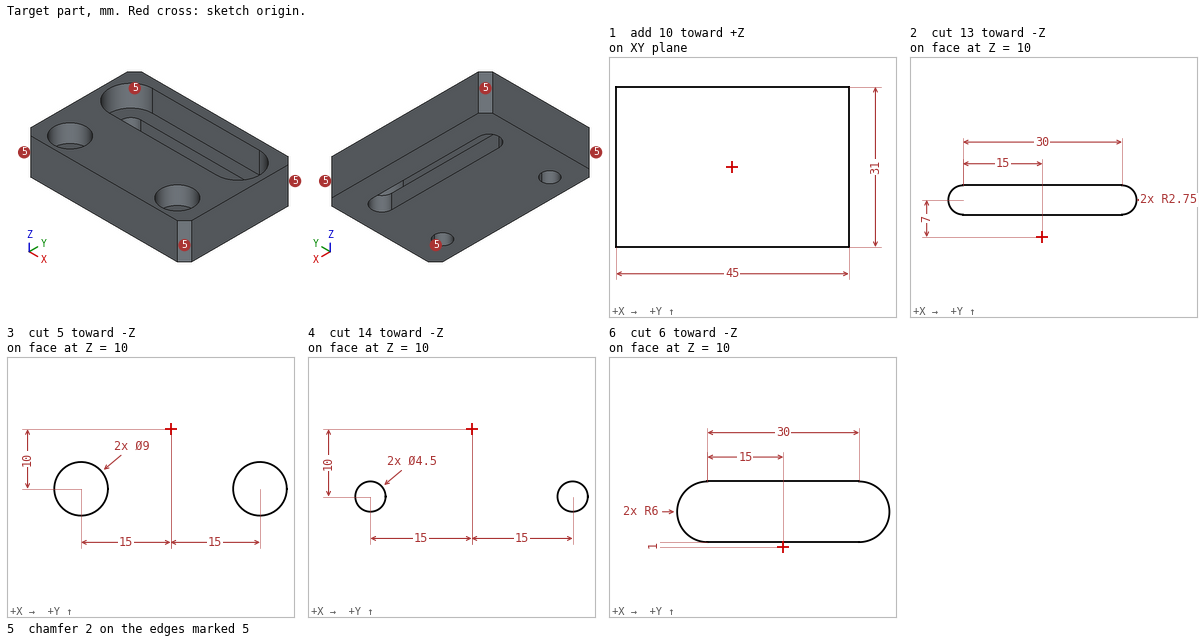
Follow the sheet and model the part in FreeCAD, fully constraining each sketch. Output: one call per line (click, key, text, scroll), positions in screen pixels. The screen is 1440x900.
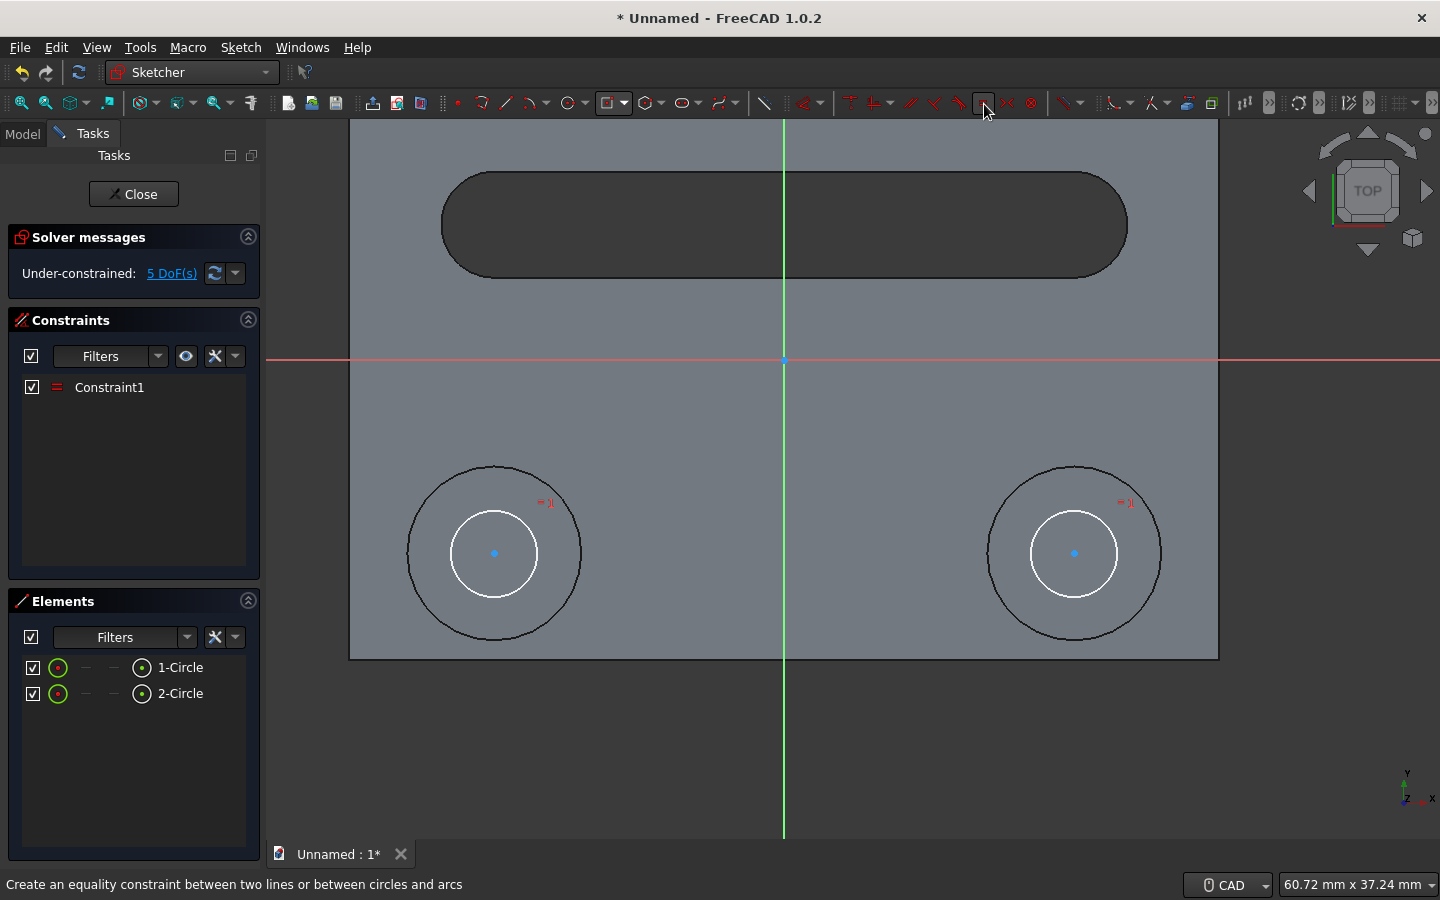
click(494, 554)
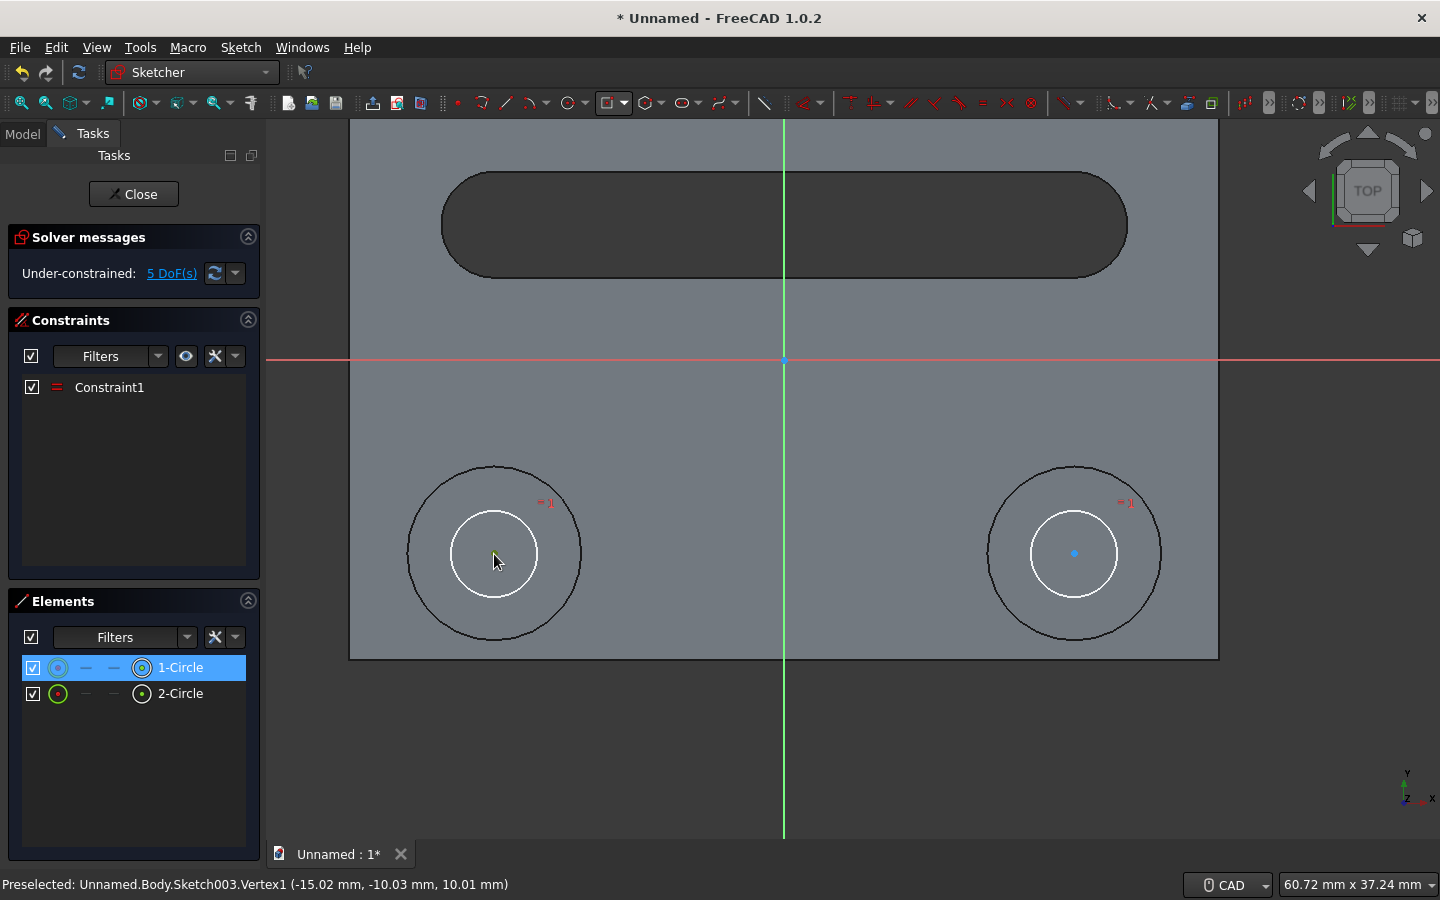
click(1074, 554)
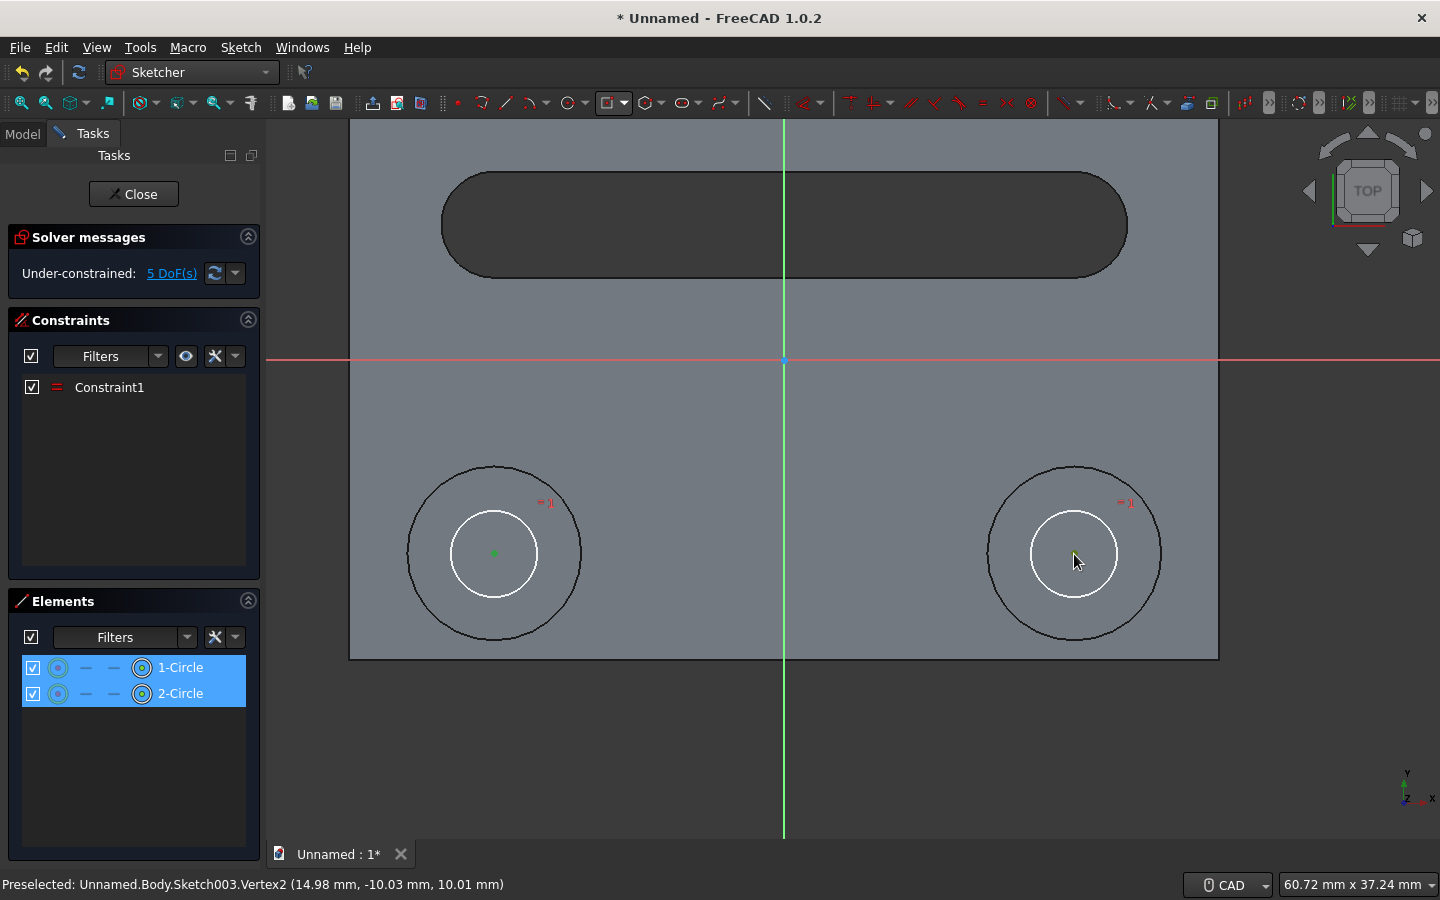
key(h)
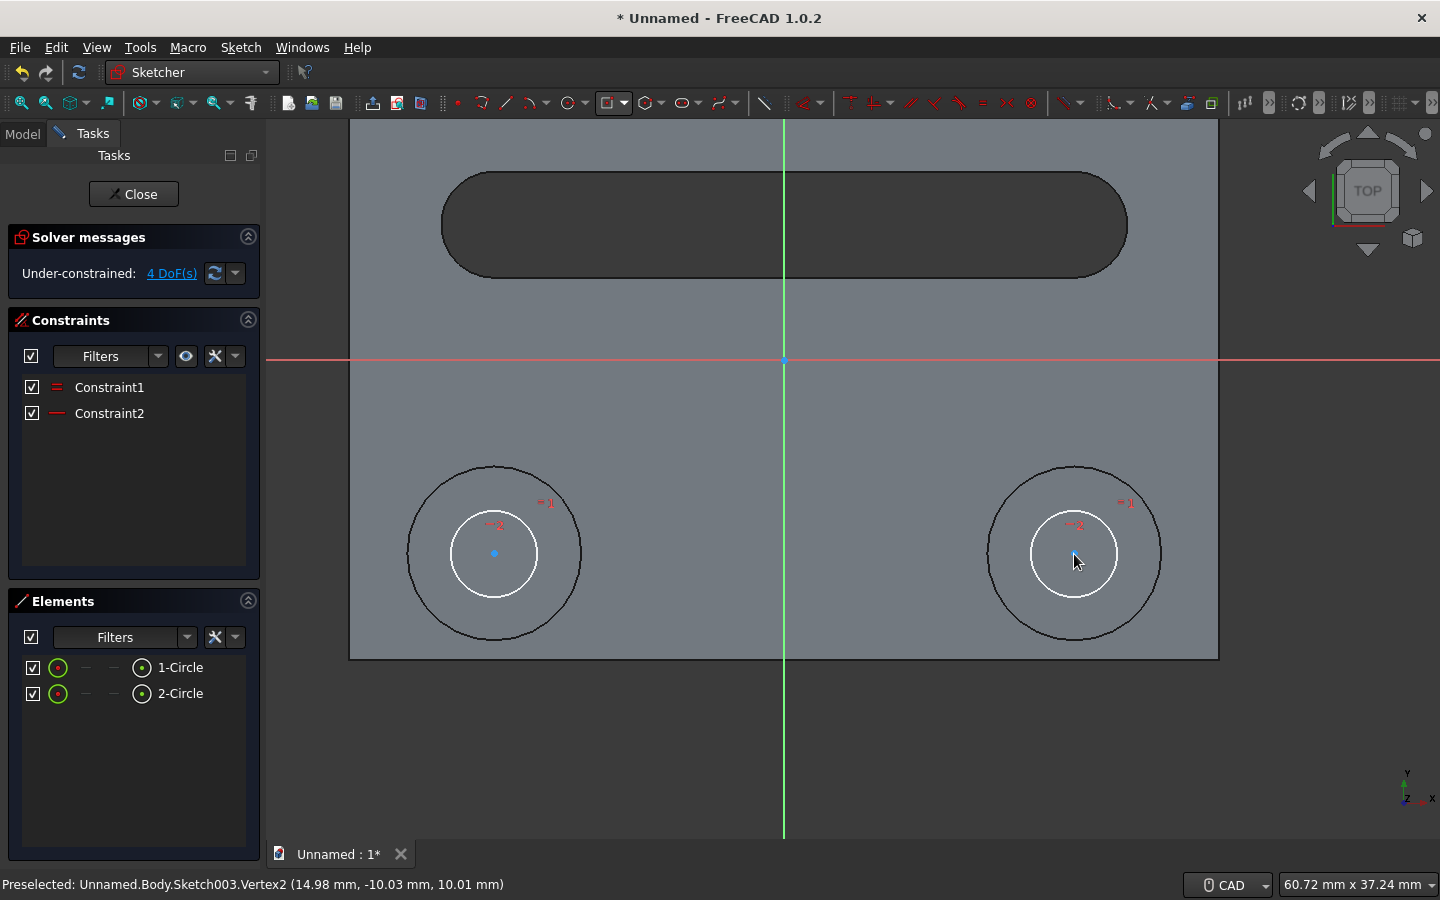
click(804, 104)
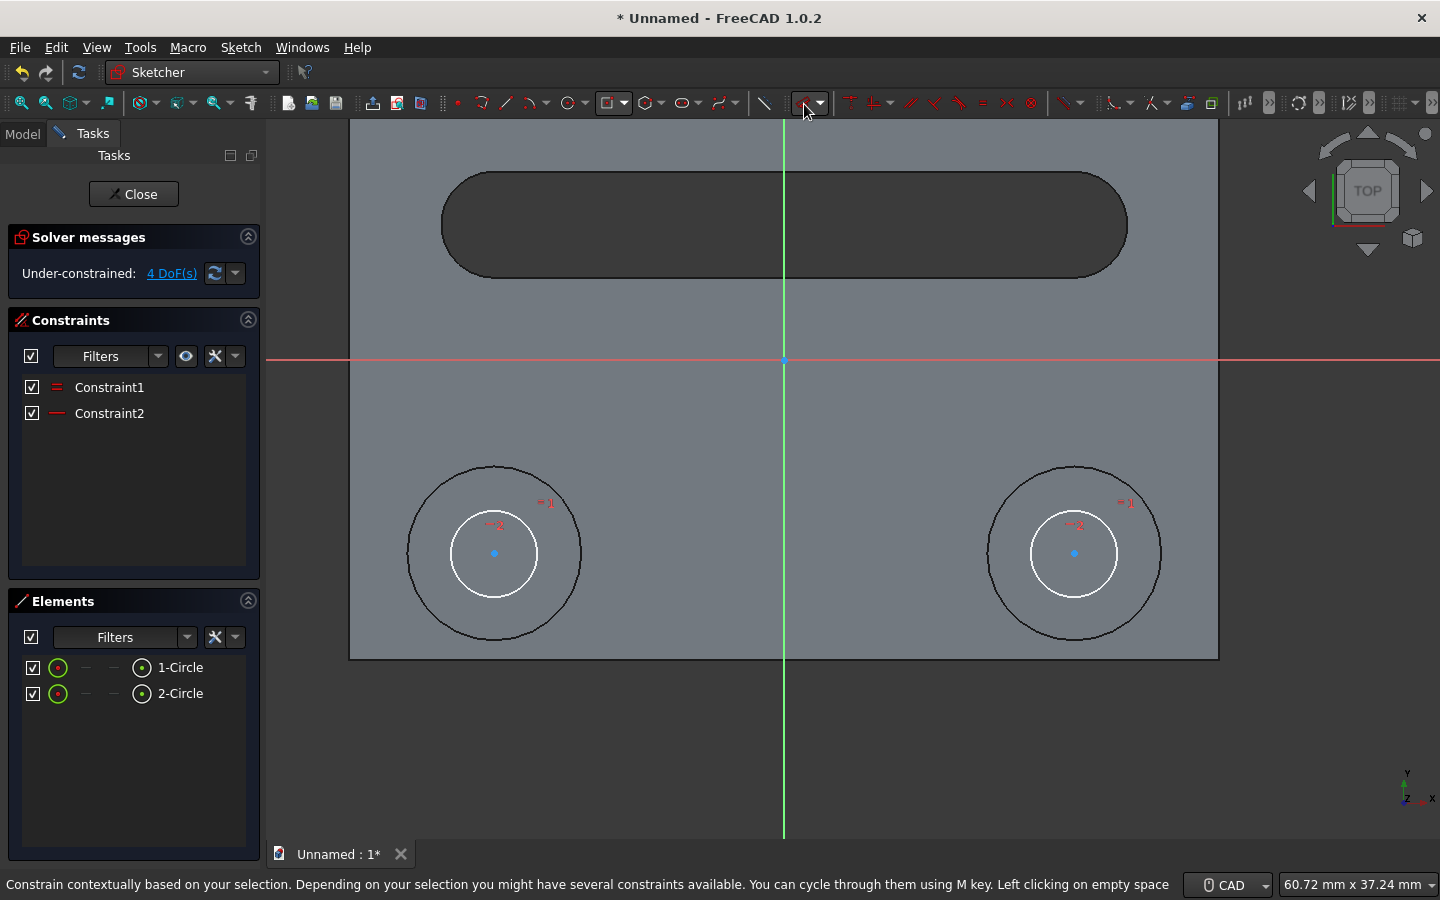
click(524, 523)
click(546, 500)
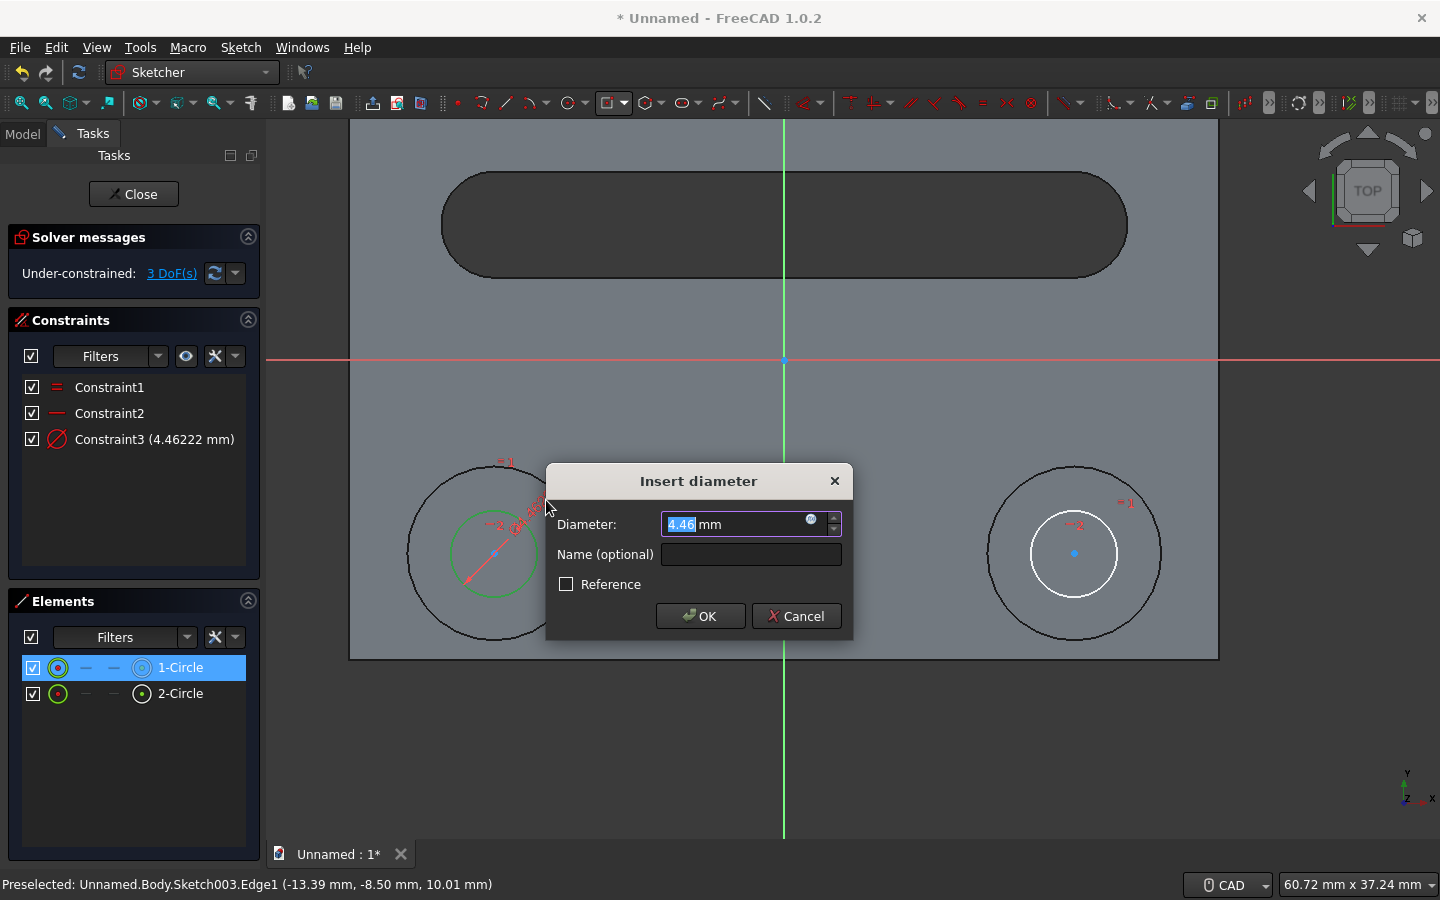
text(4.5)
key(Return)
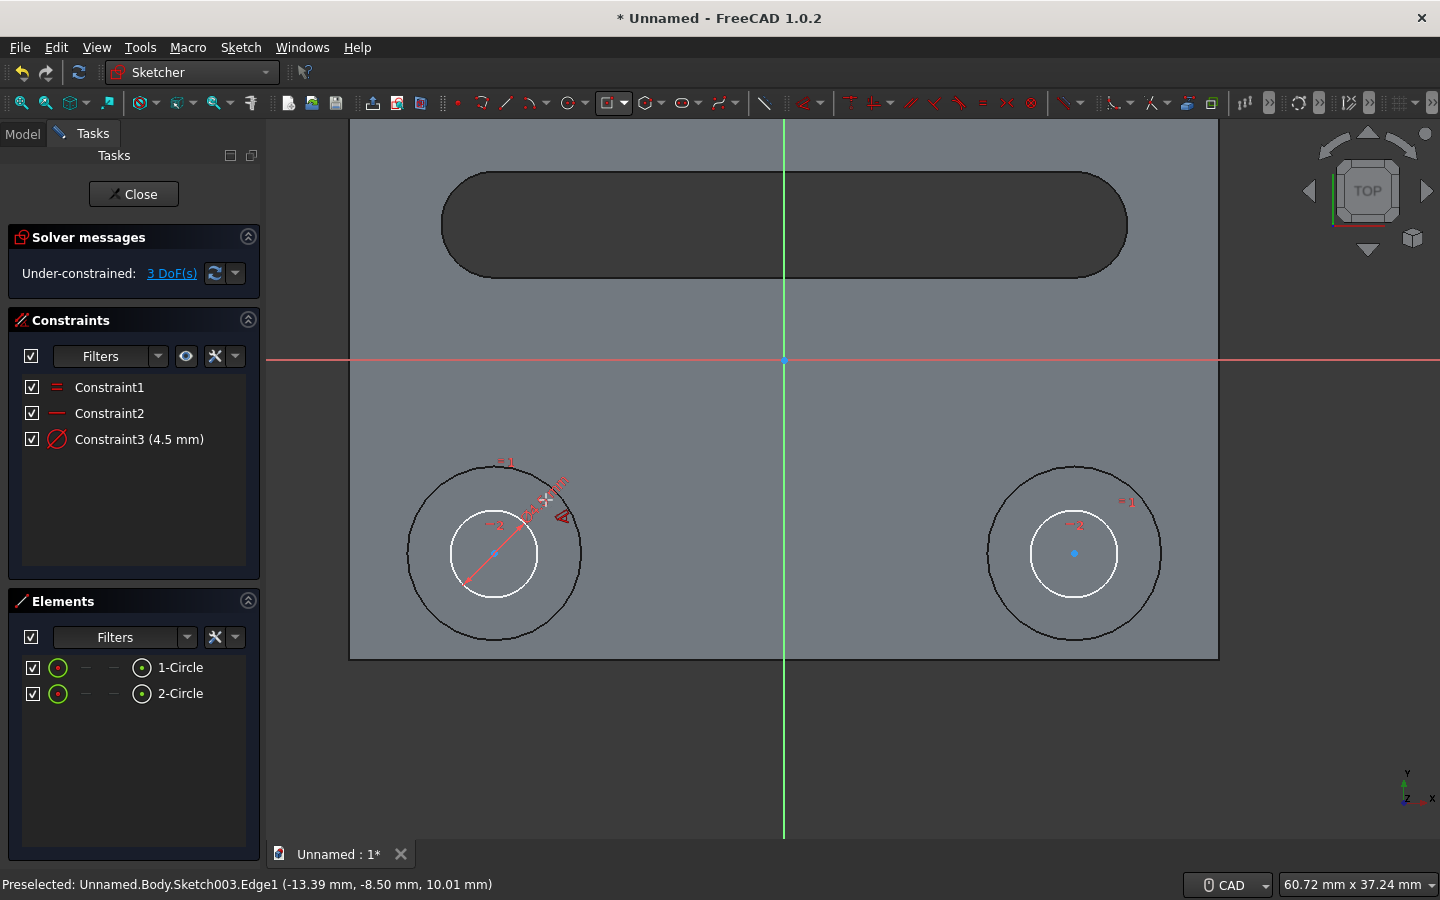
click(494, 554)
click(639, 326)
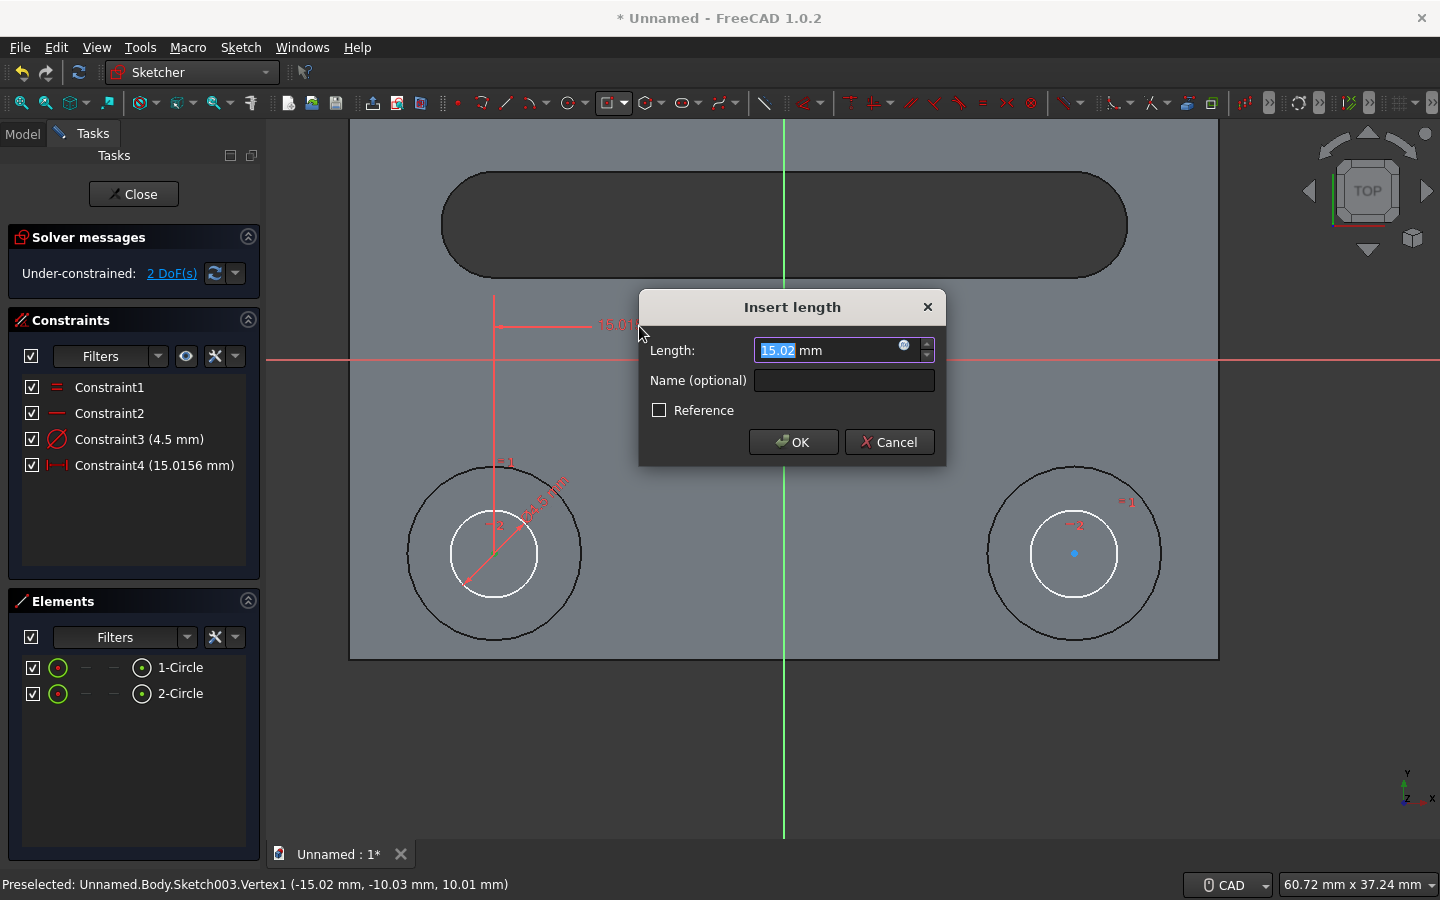
text(15)
key(Return)